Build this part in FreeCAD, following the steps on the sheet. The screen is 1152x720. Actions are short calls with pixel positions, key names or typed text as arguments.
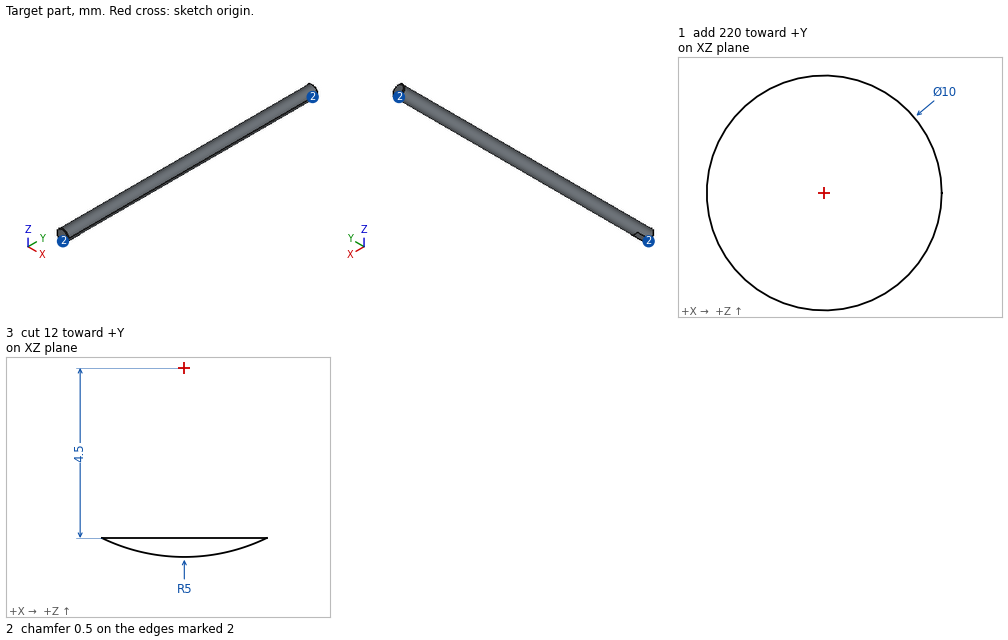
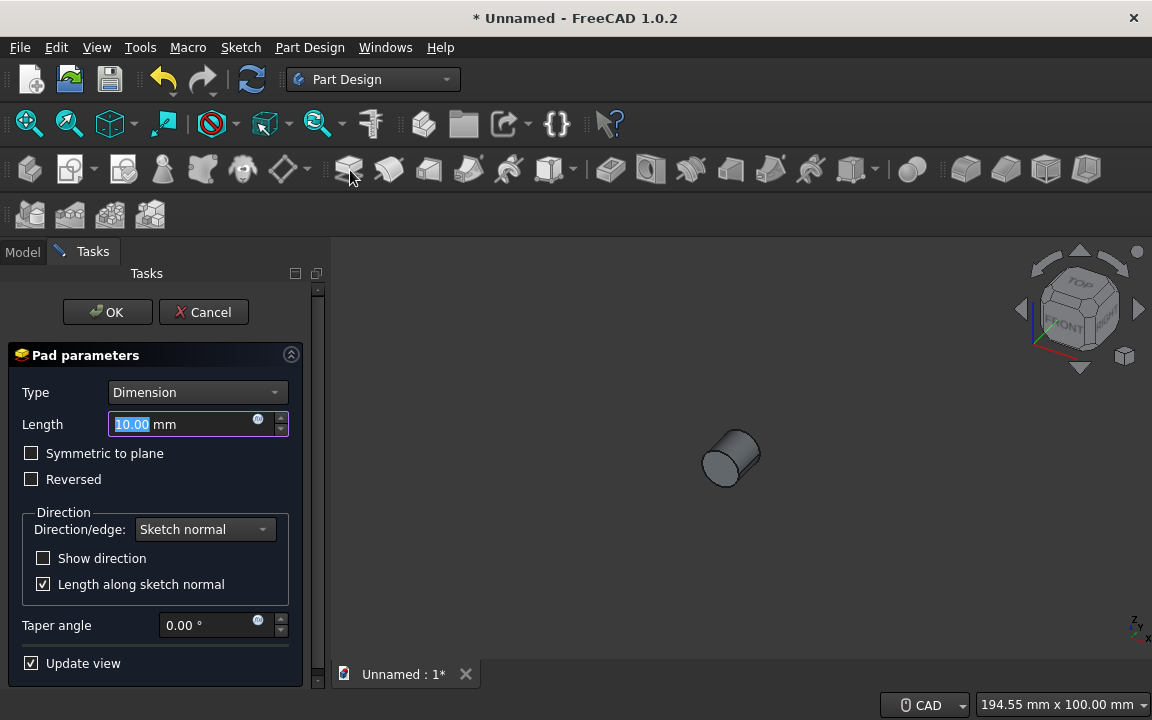
text(220)
key(Tab)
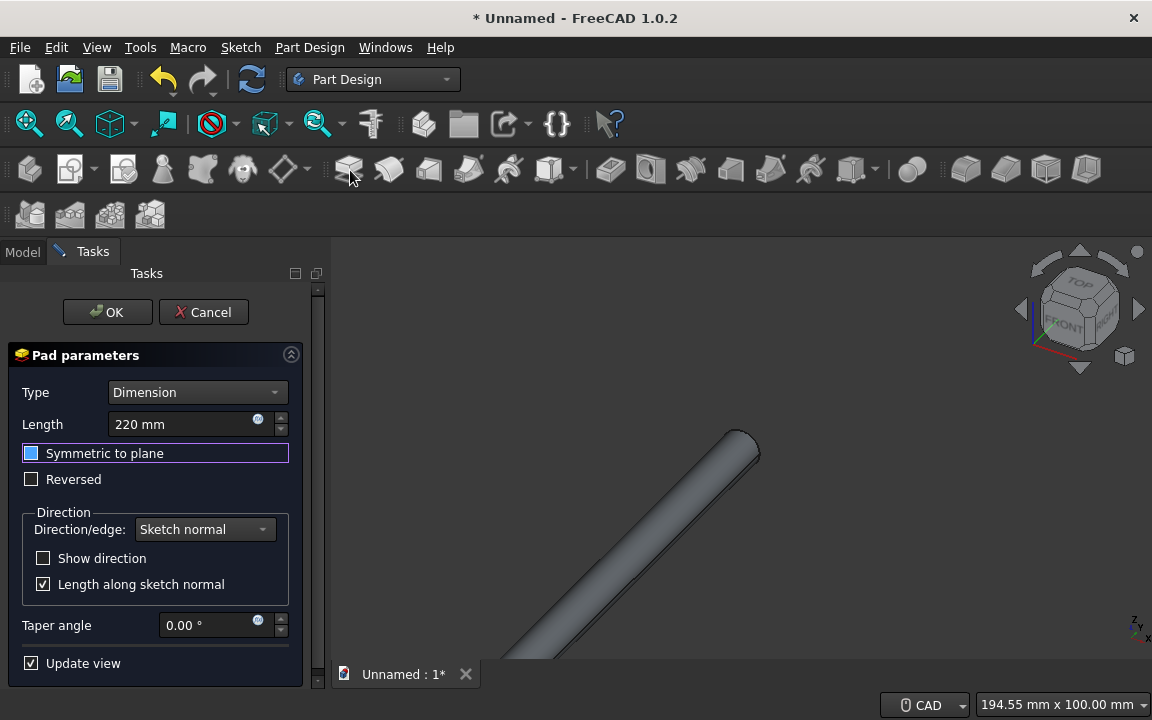
click(30, 479)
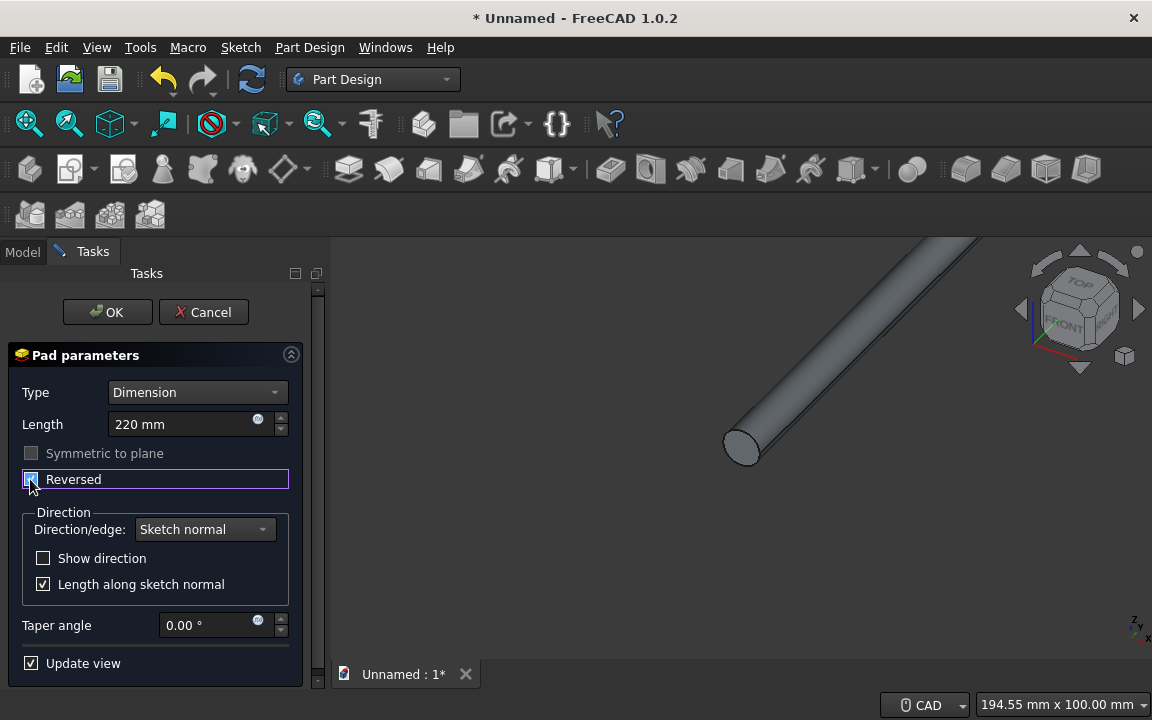
click(108, 312)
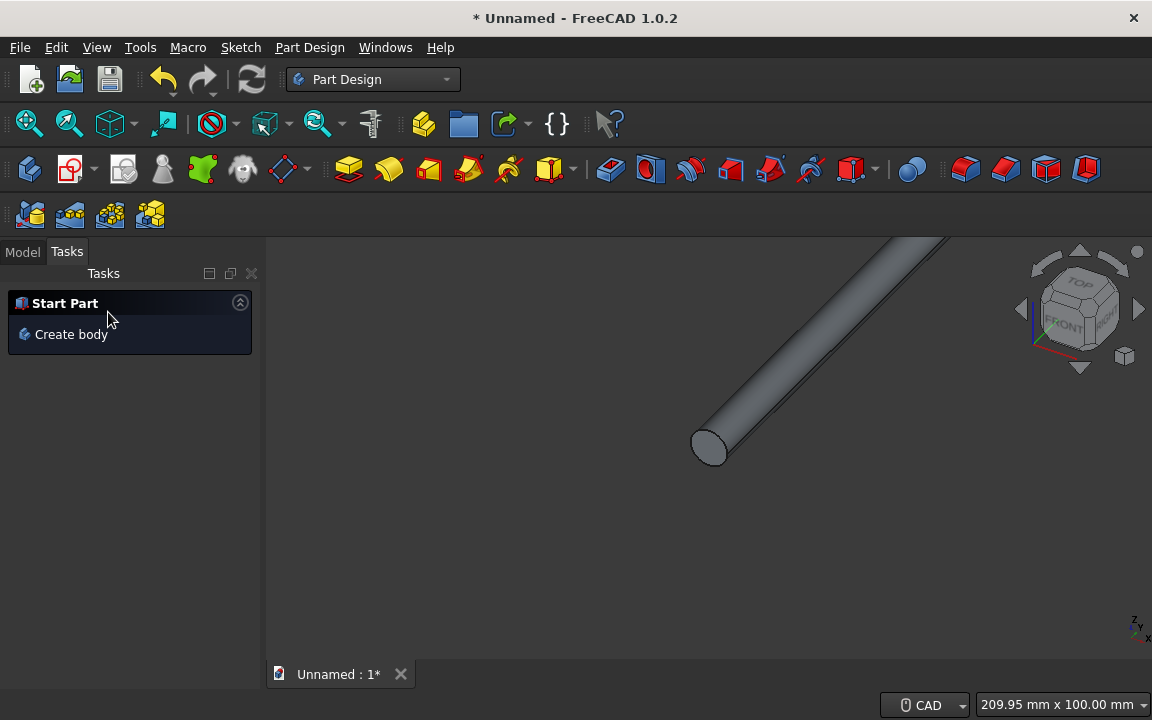
click(30, 124)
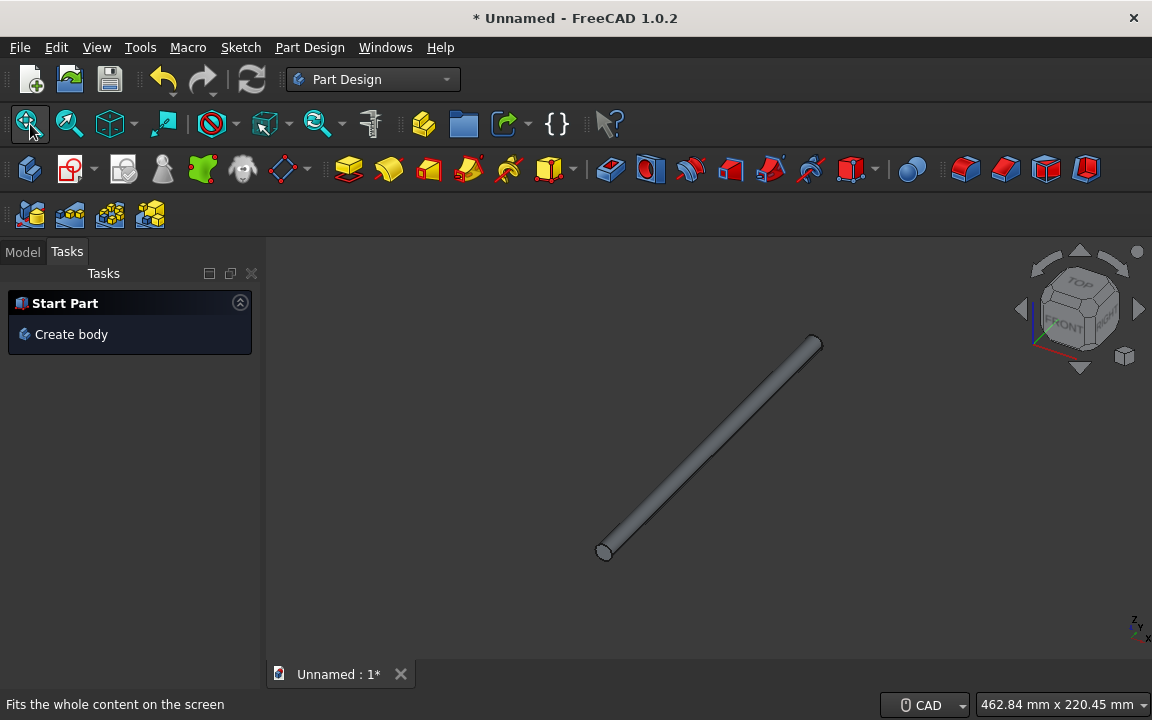
click(595, 549)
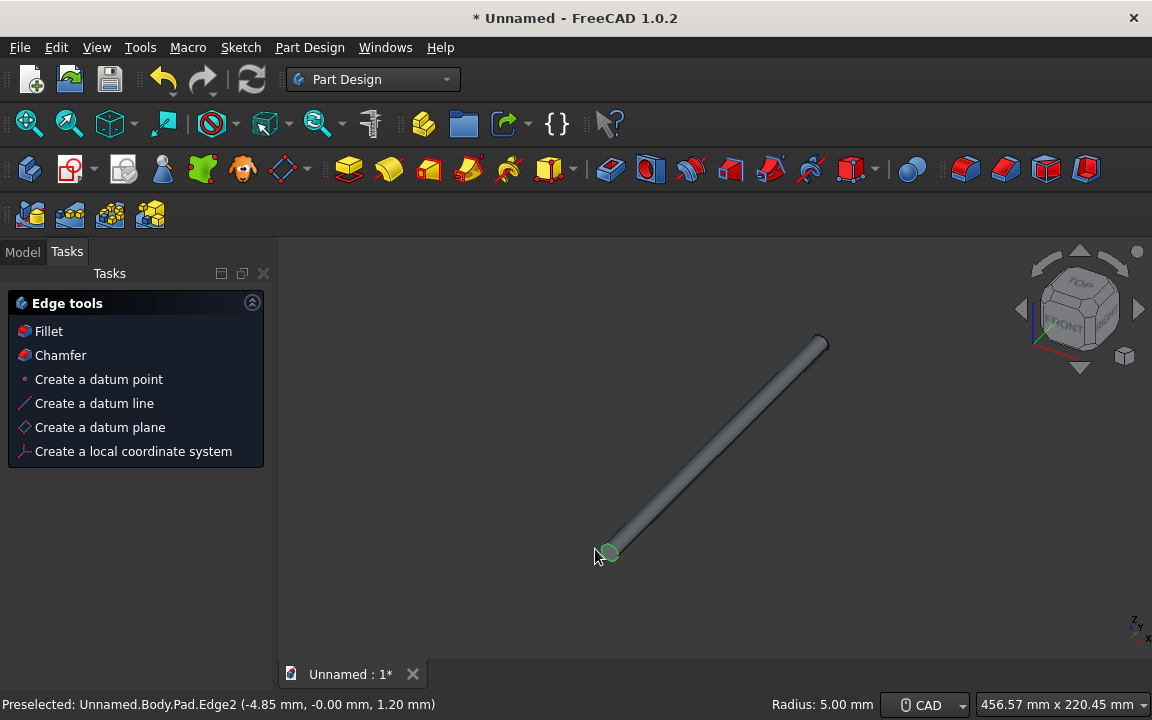
click(818, 334, ctrl)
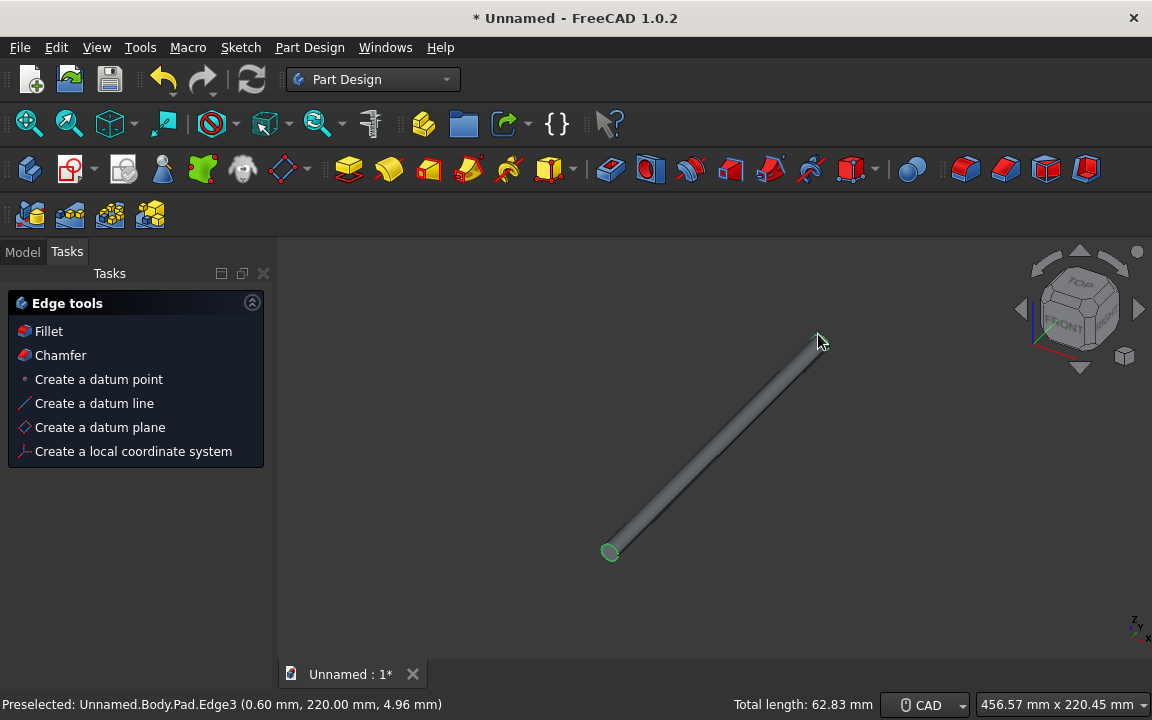
click(1006, 170)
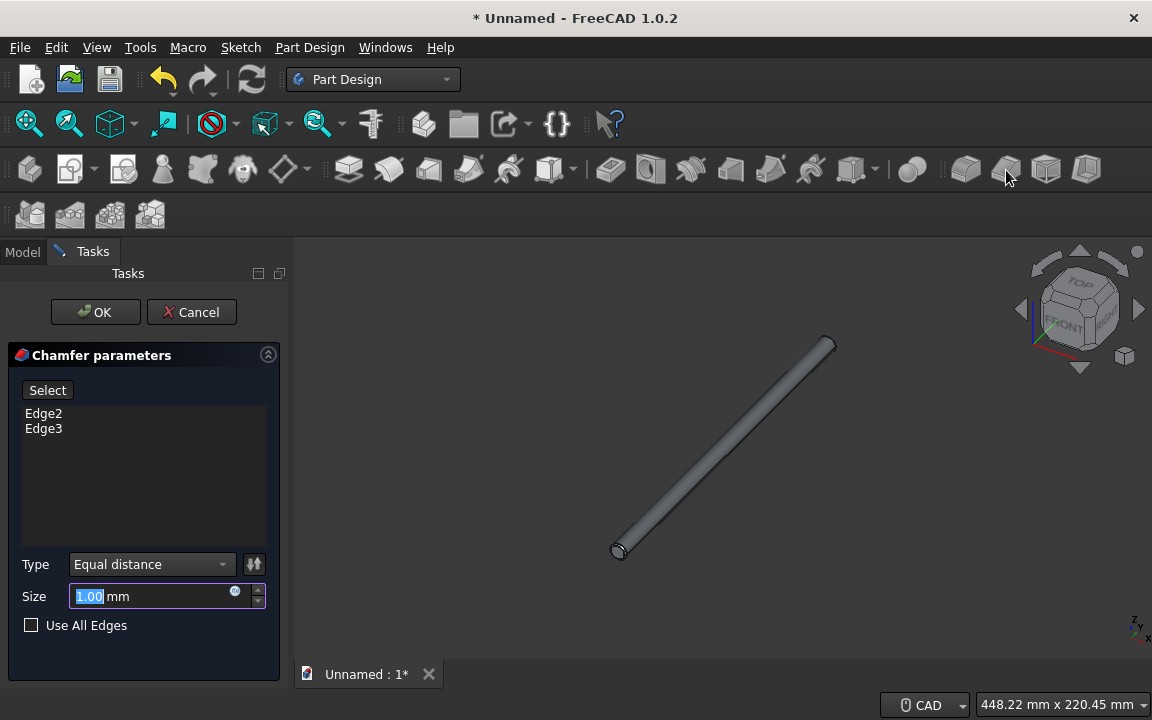
text(0.5)
key(Tab)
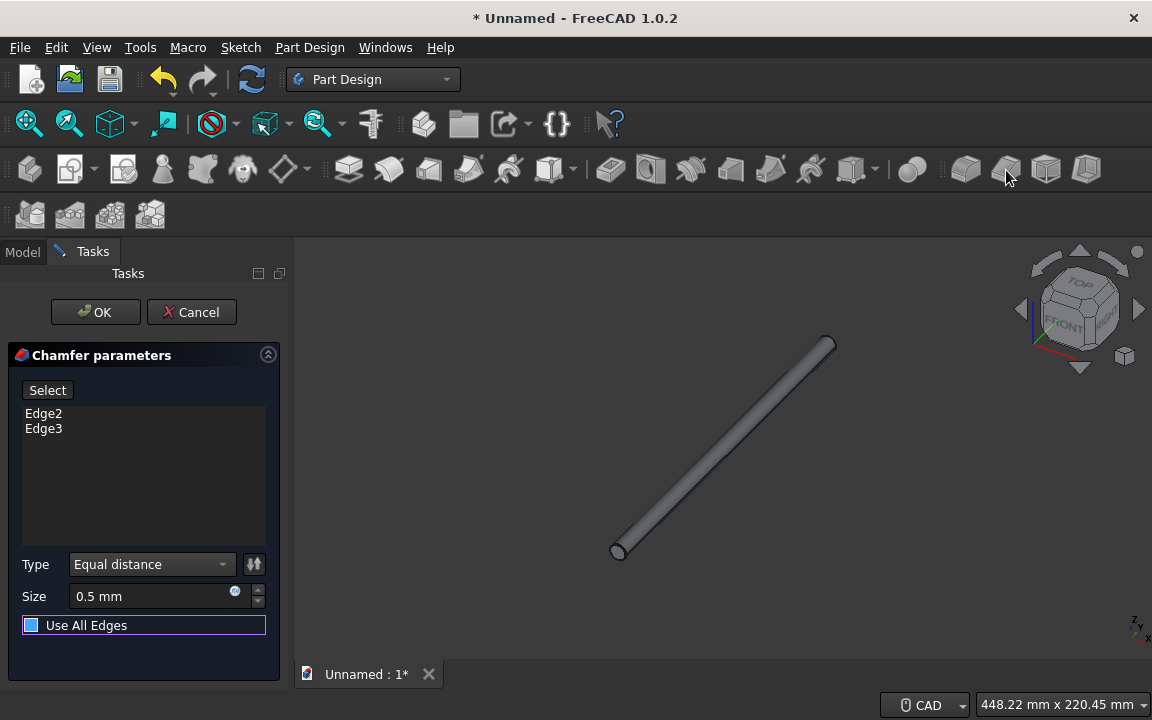
click(96, 312)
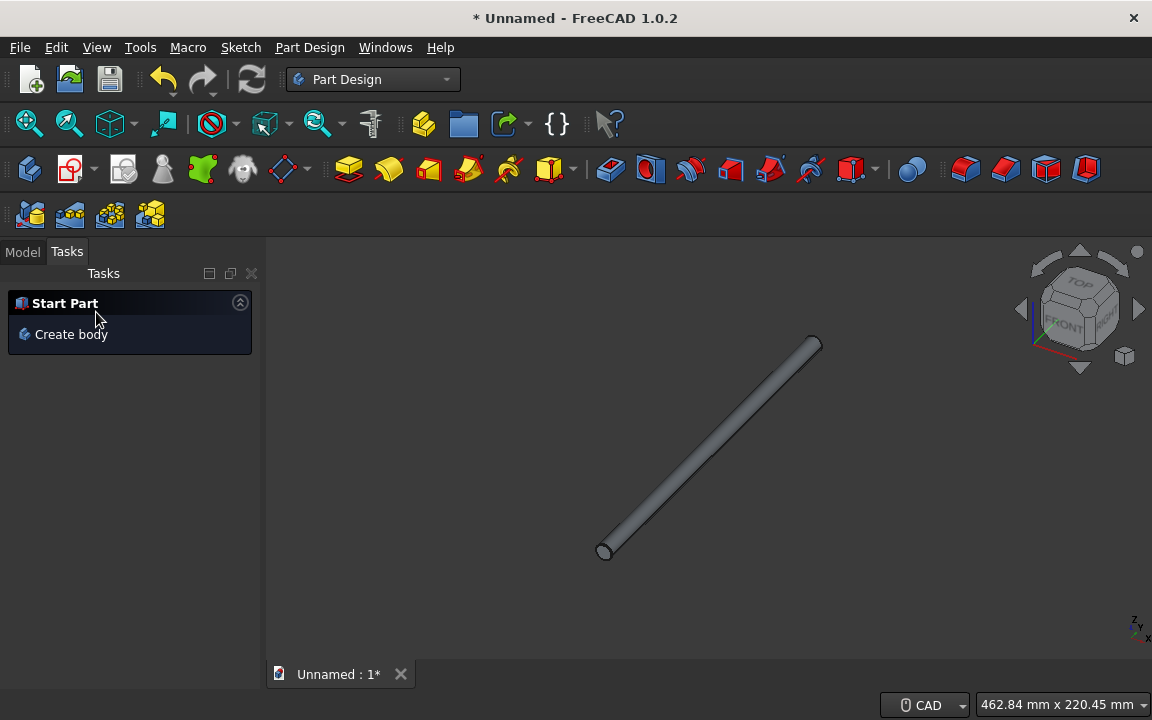
key(0)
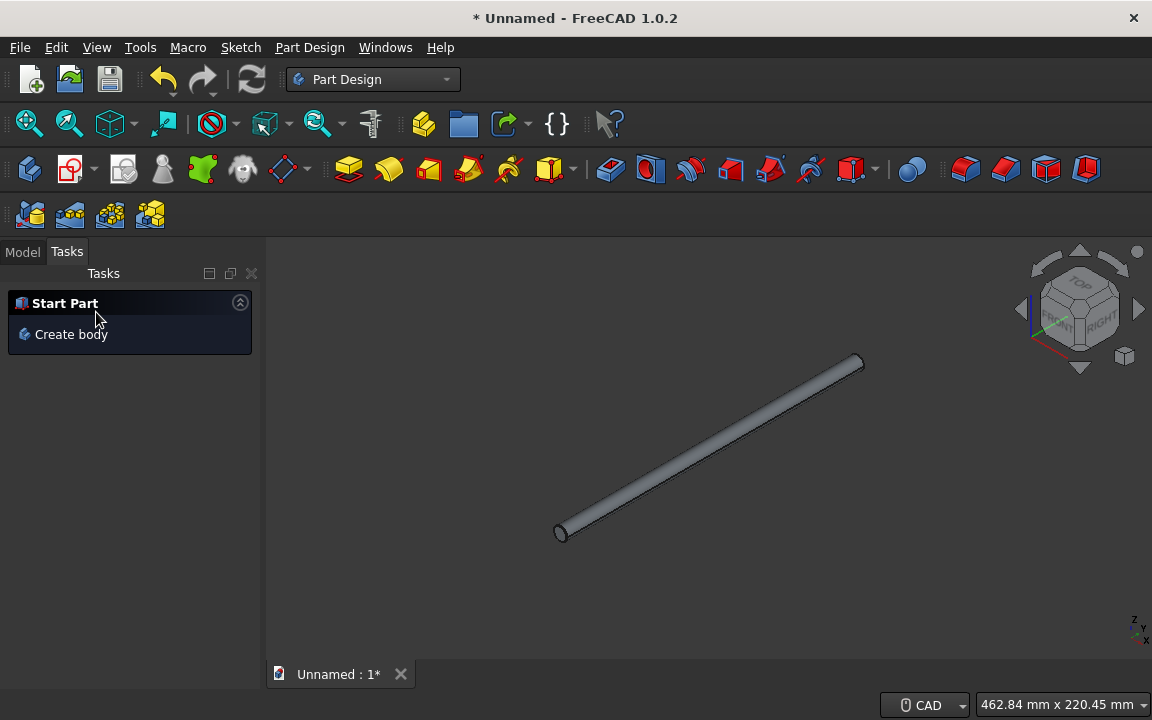
key(1)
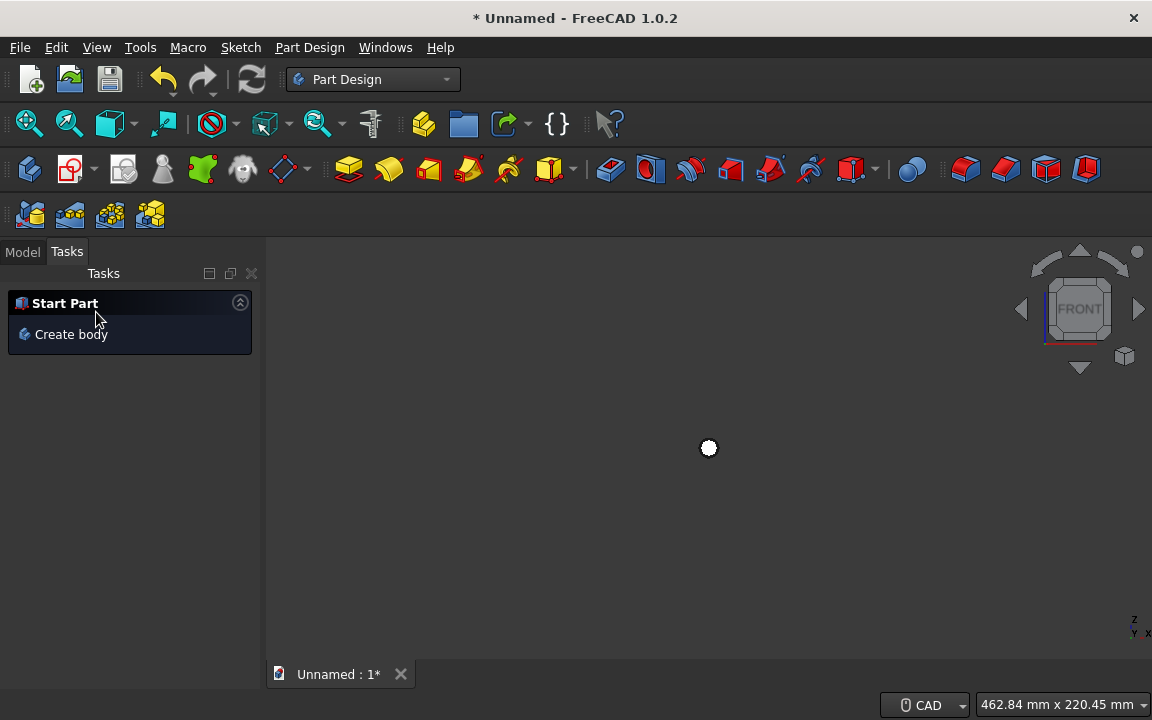
click(30, 124)